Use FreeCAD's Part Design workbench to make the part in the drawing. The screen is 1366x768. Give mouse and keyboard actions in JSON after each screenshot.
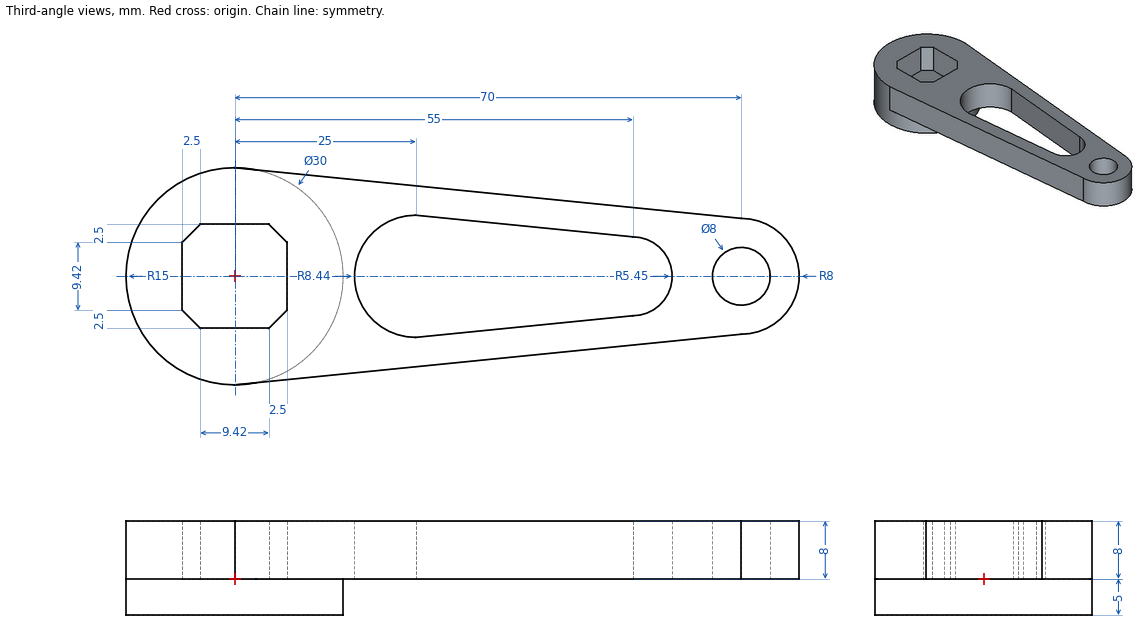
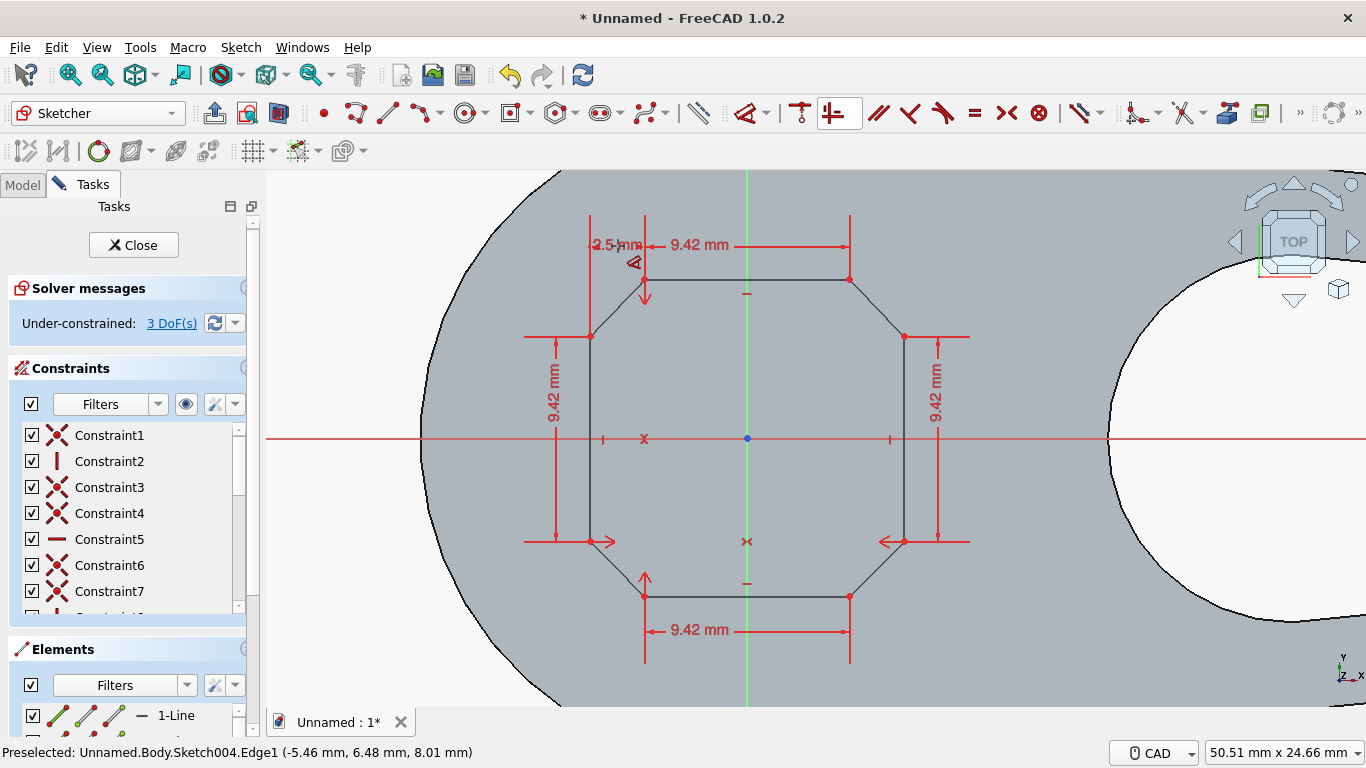
{"action": "left_click", "coordinate": [628, 297]}
{"action": "left_click", "coordinate": [556, 308]}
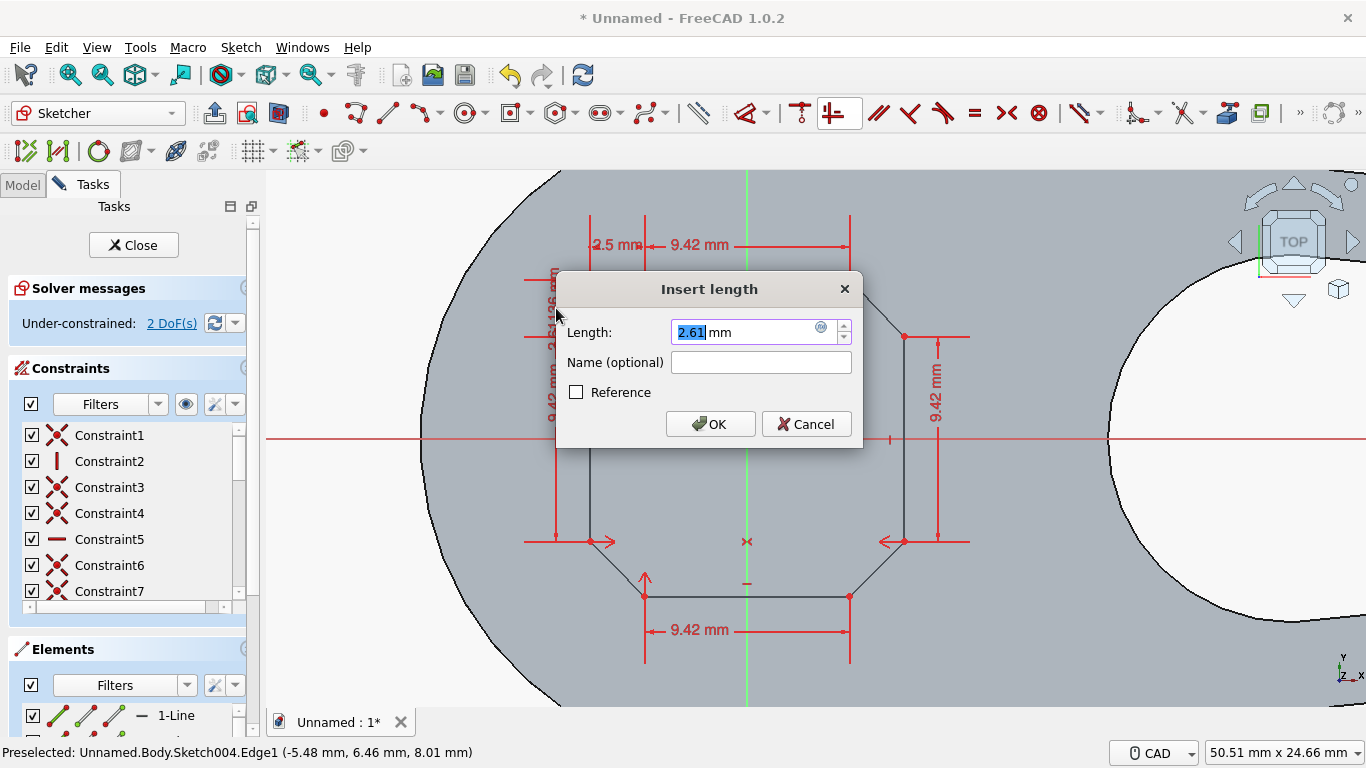
{"action": "type", "text": "2.5"}
{"action": "key", "text": "Return"}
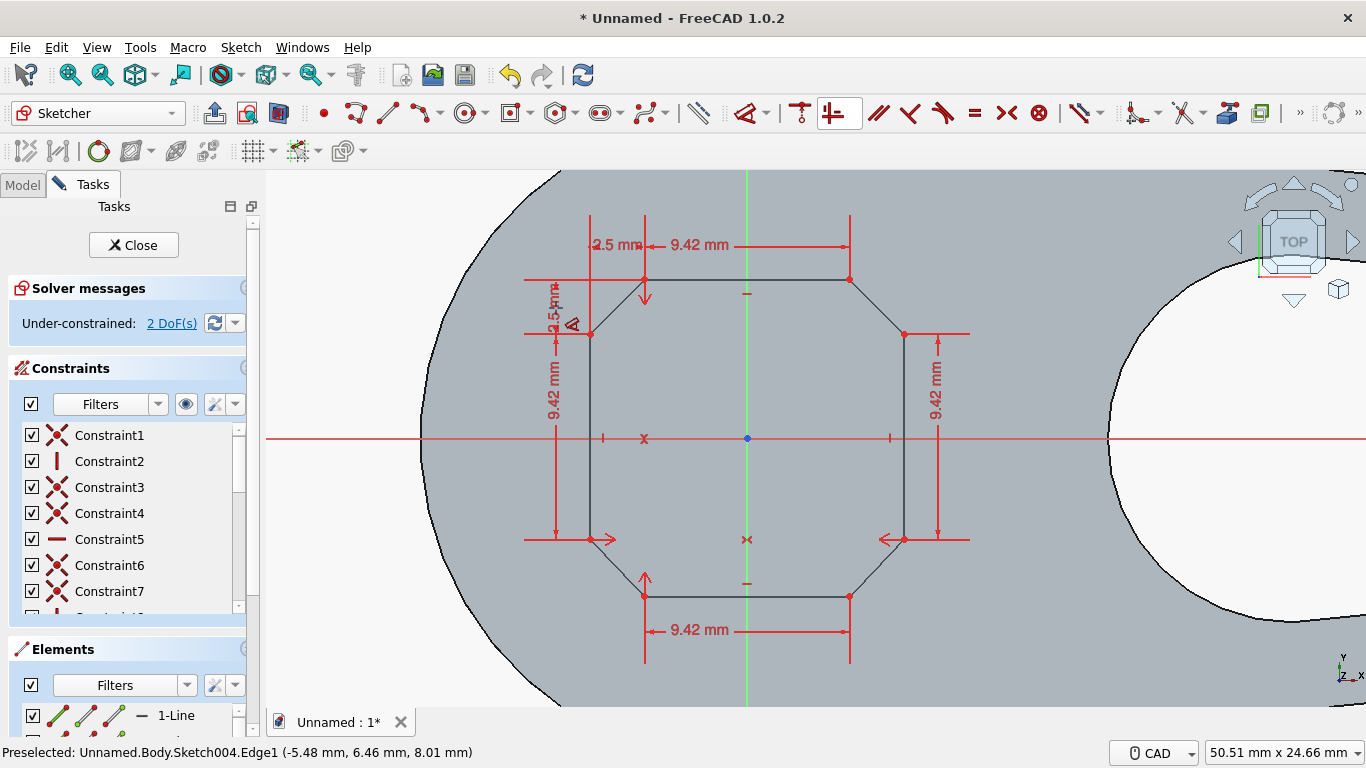
{"action": "left_click", "coordinate": [607, 557]}
{"action": "left_click", "coordinate": [556, 568]}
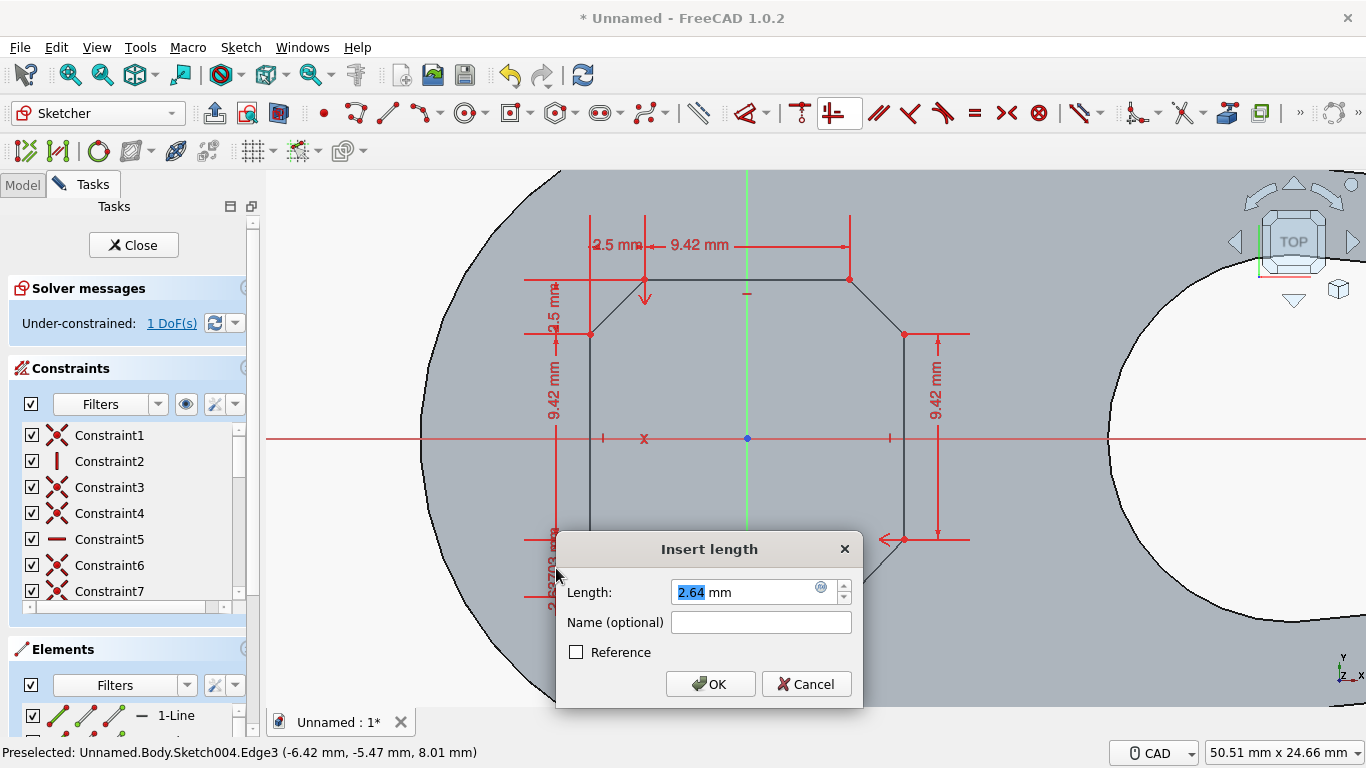
{"action": "type", "text": "2.5"}
{"action": "key", "text": "Return"}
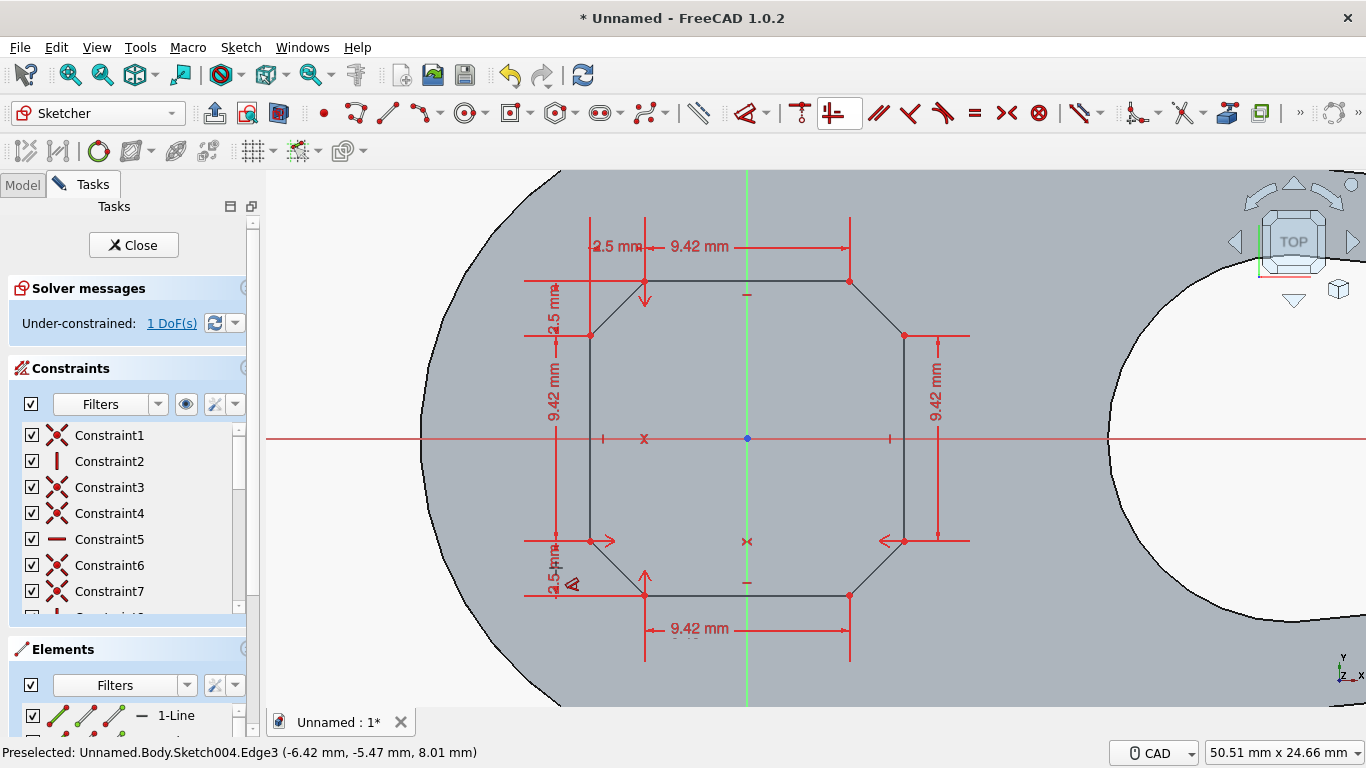
{"action": "left_click", "coordinate": [866, 579]}
{"action": "left_click", "coordinate": [877, 630]}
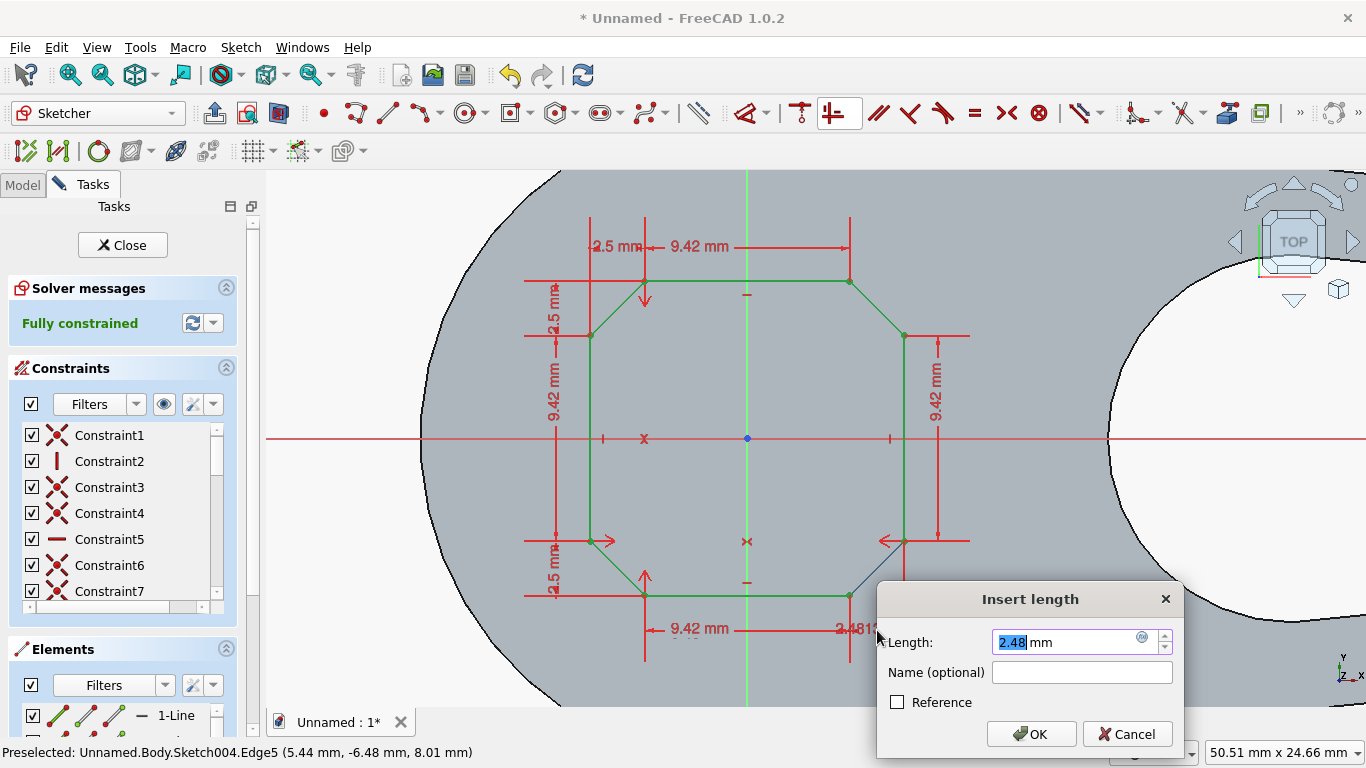
{"action": "type", "text": "2.5"}
{"action": "key", "text": "Return"}
{"action": "key", "text": "Escape"}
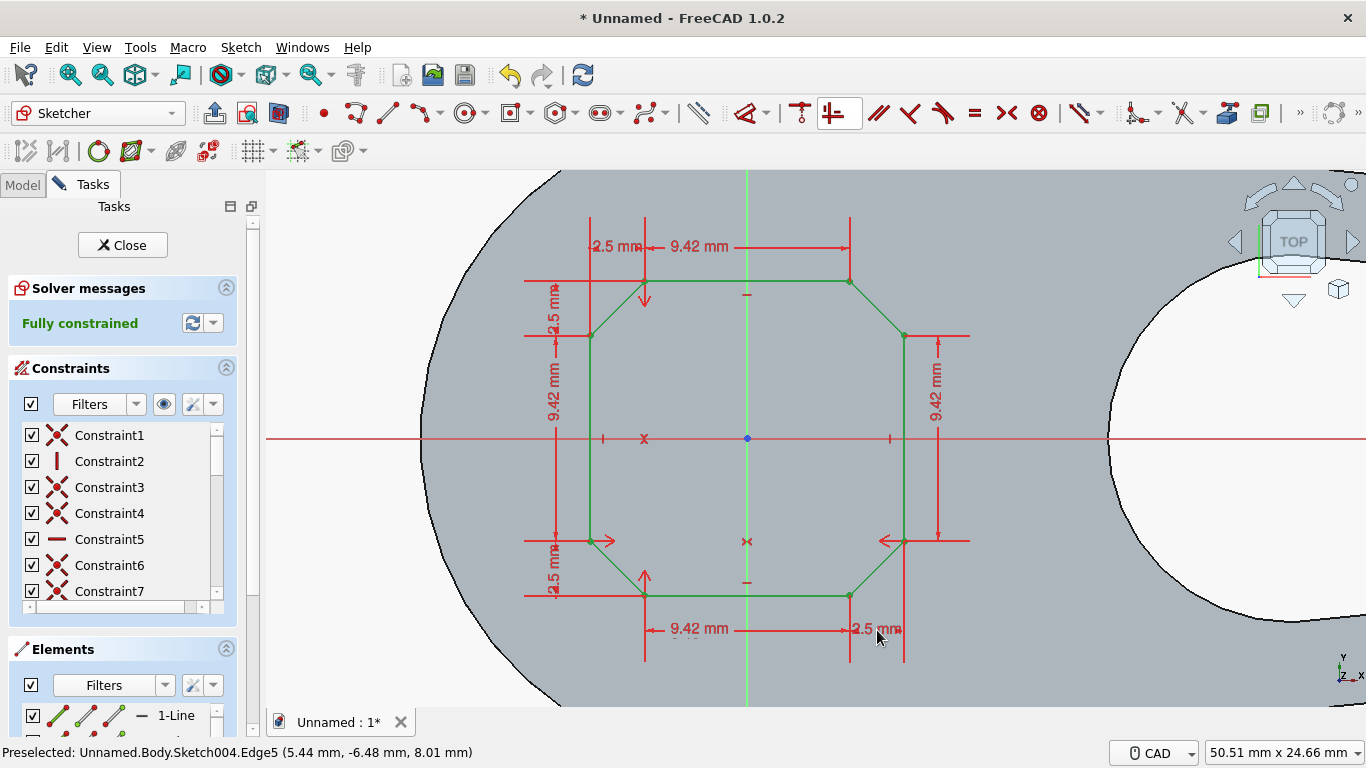
{"action": "left_click", "coordinate": [123, 245]}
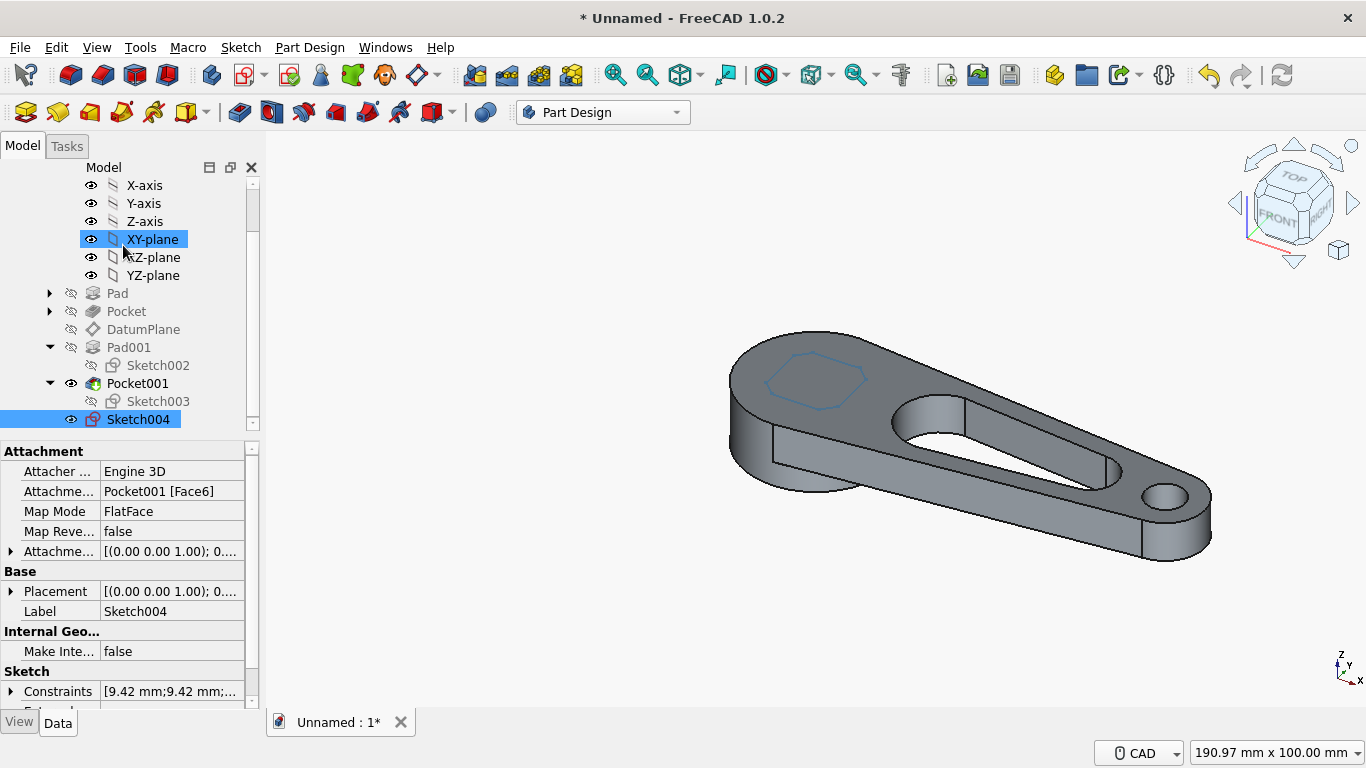
{"action": "left_click", "coordinate": [240, 112]}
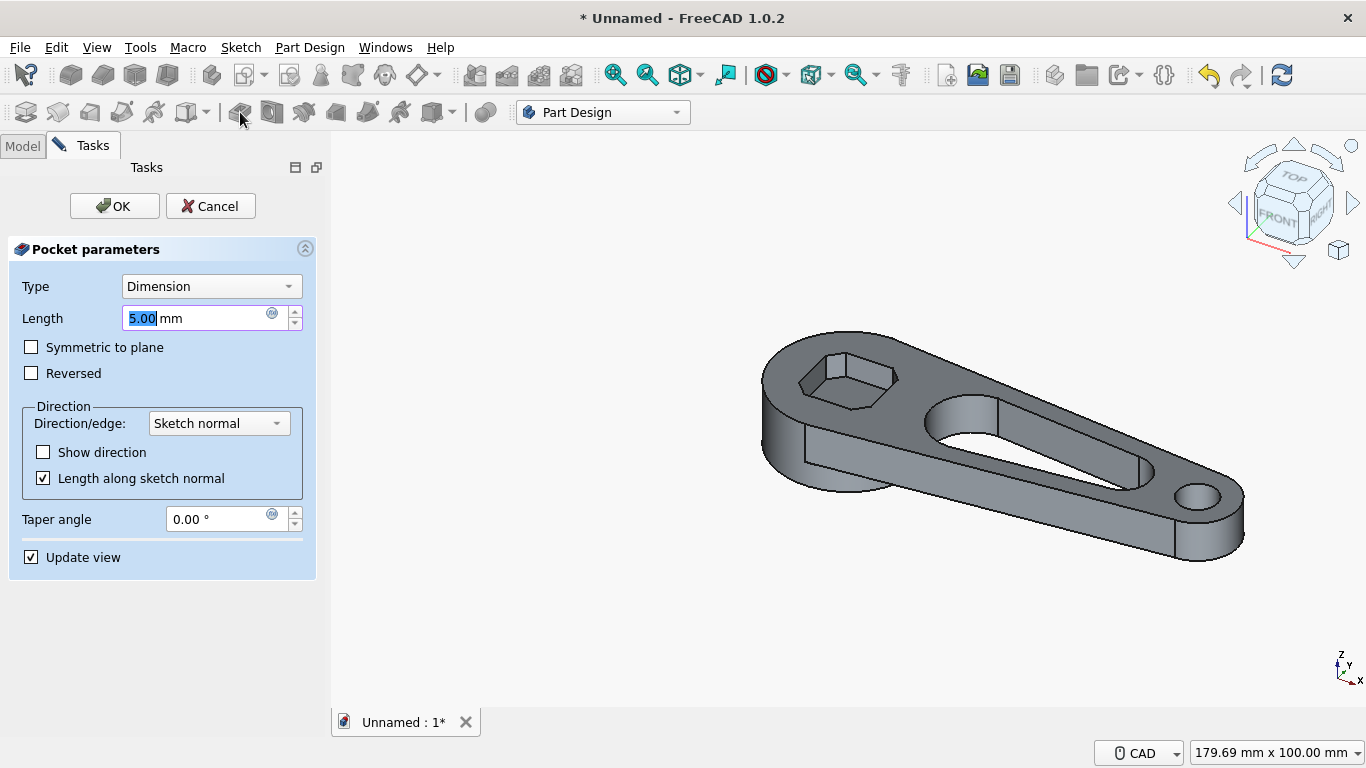
{"action": "type", "text": "8"}
{"action": "key", "text": "Tab"}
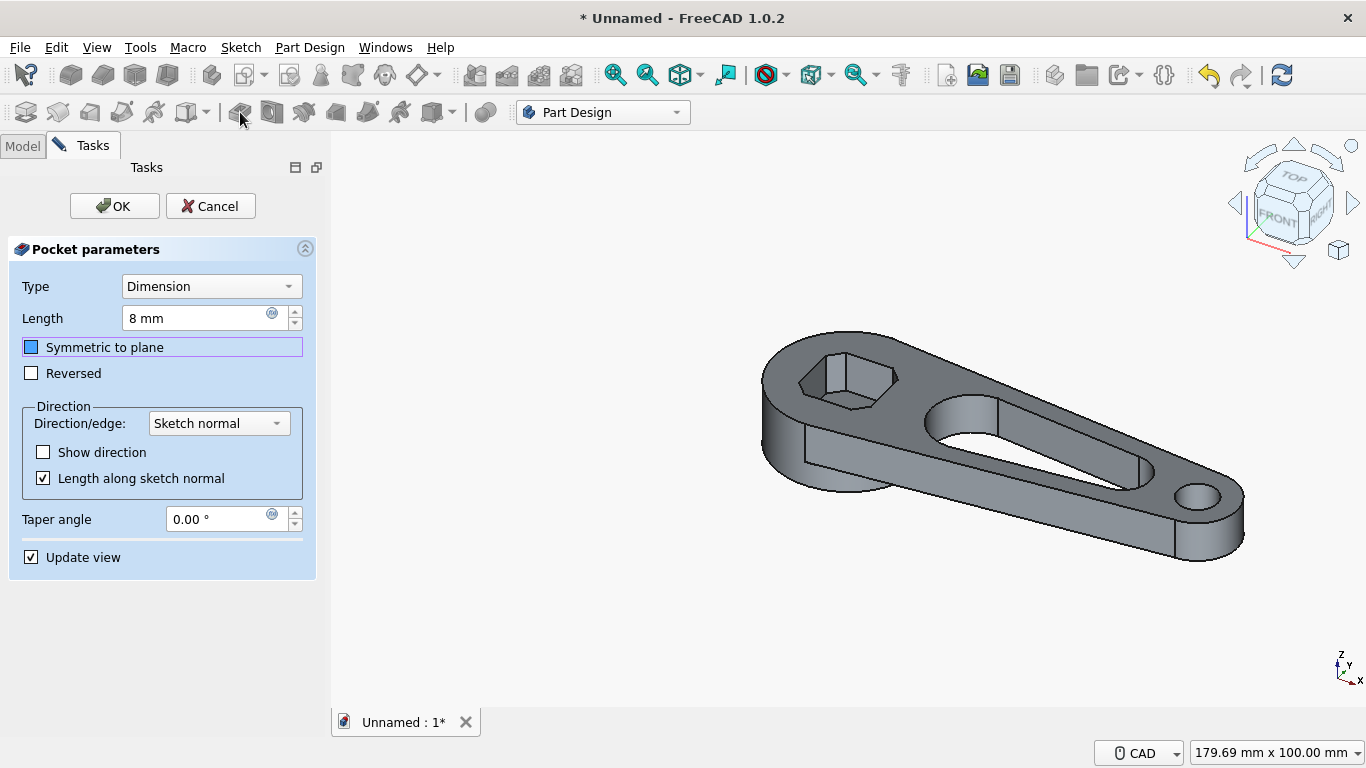
{"action": "left_click", "coordinate": [115, 206]}